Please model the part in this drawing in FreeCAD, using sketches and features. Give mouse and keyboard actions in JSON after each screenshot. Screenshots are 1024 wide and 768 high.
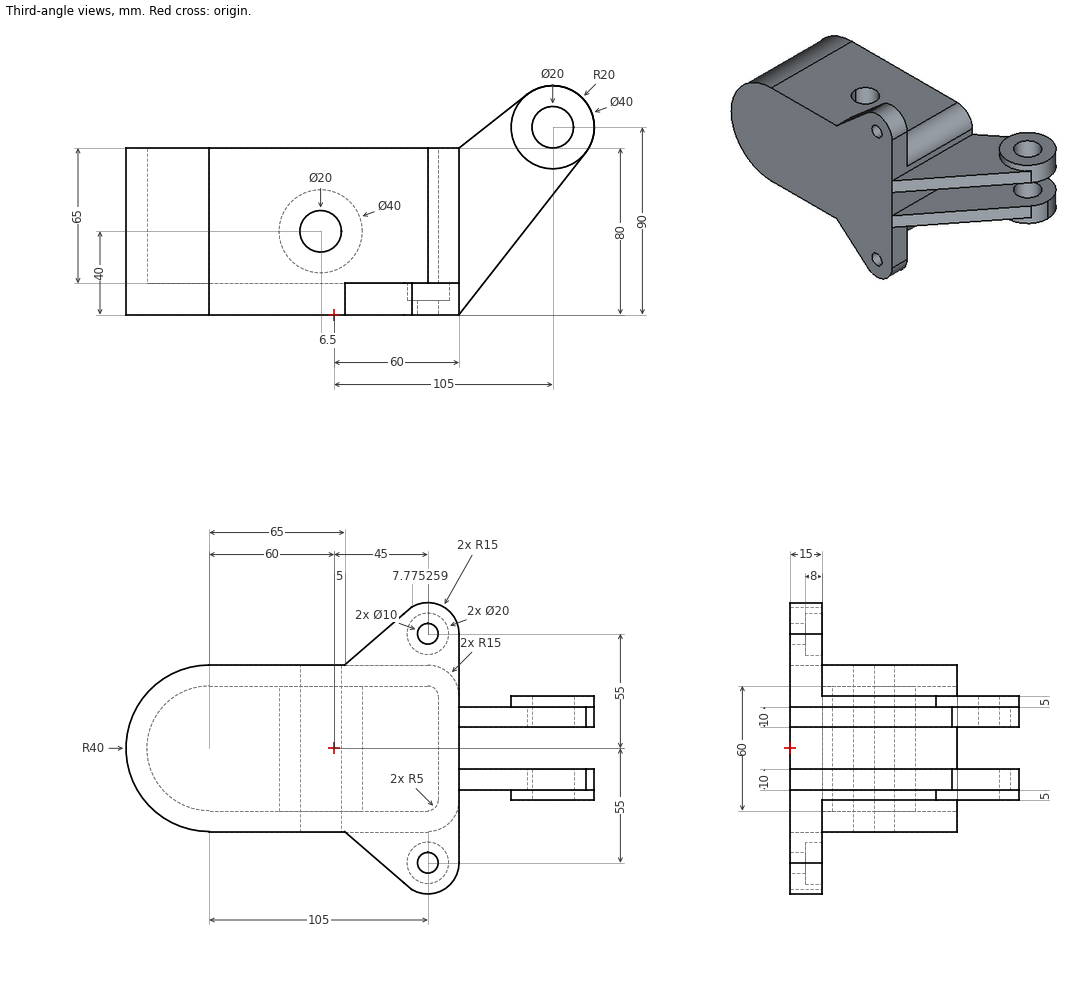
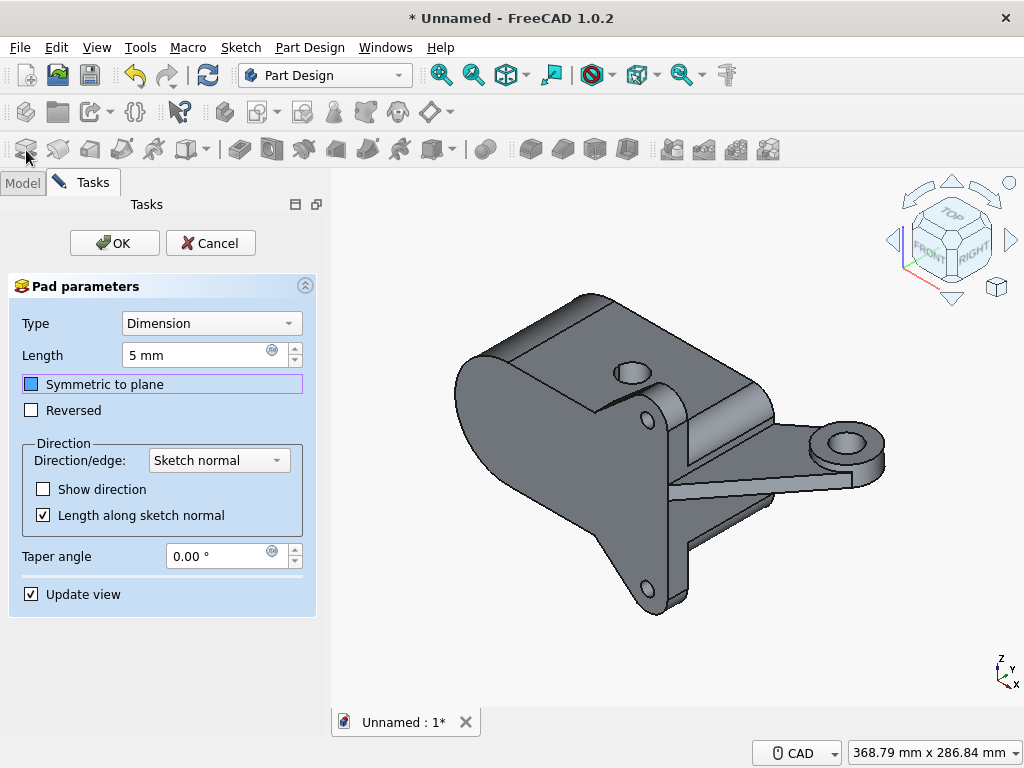
{"action": "left_click", "coordinate": [115, 243]}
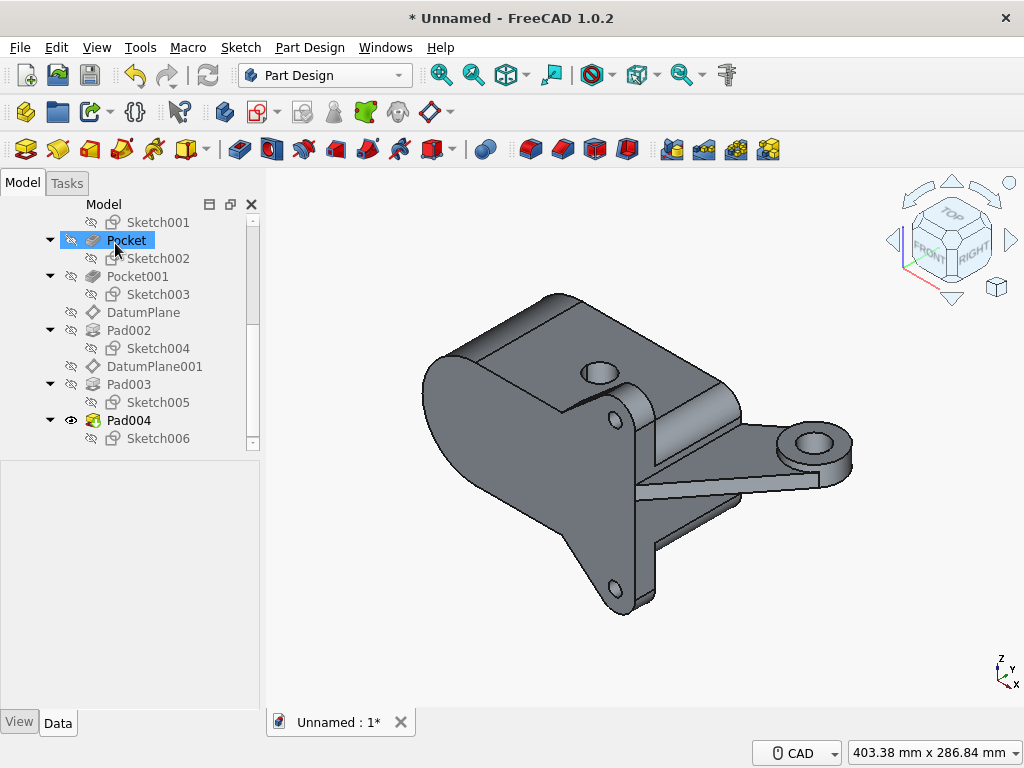
{"action": "scroll", "coordinate": [160, 326], "scroll_direction": "down", "scroll_amount": 3}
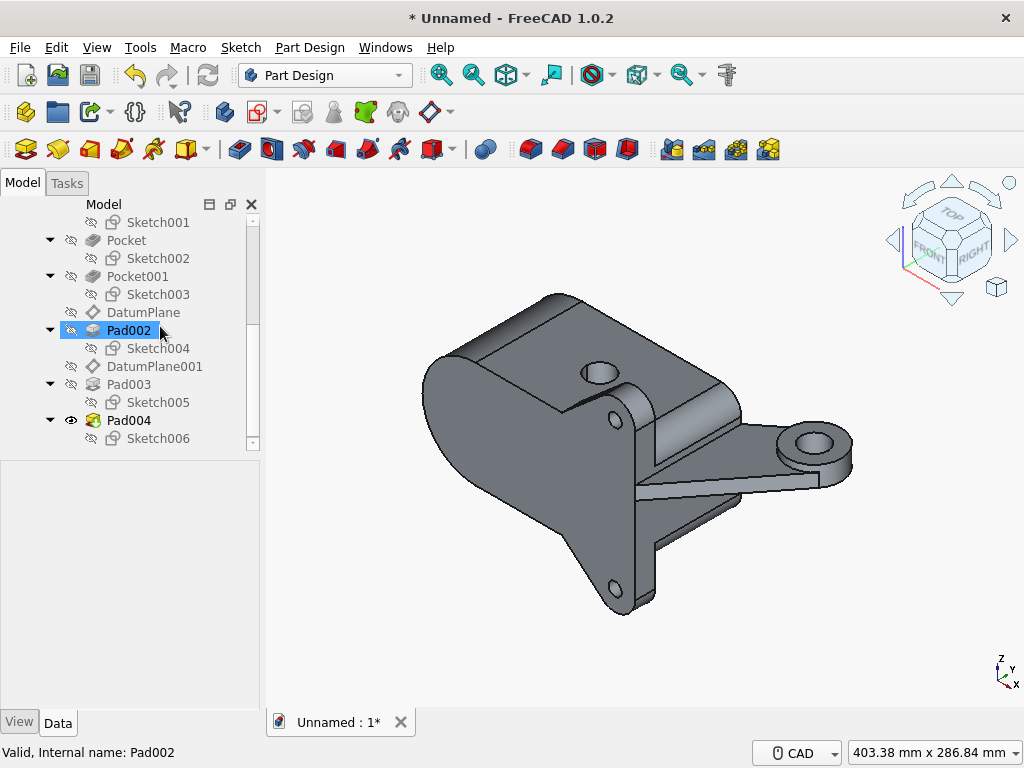
{"action": "scroll", "coordinate": [160, 326], "scroll_direction": "up", "scroll_amount": 15}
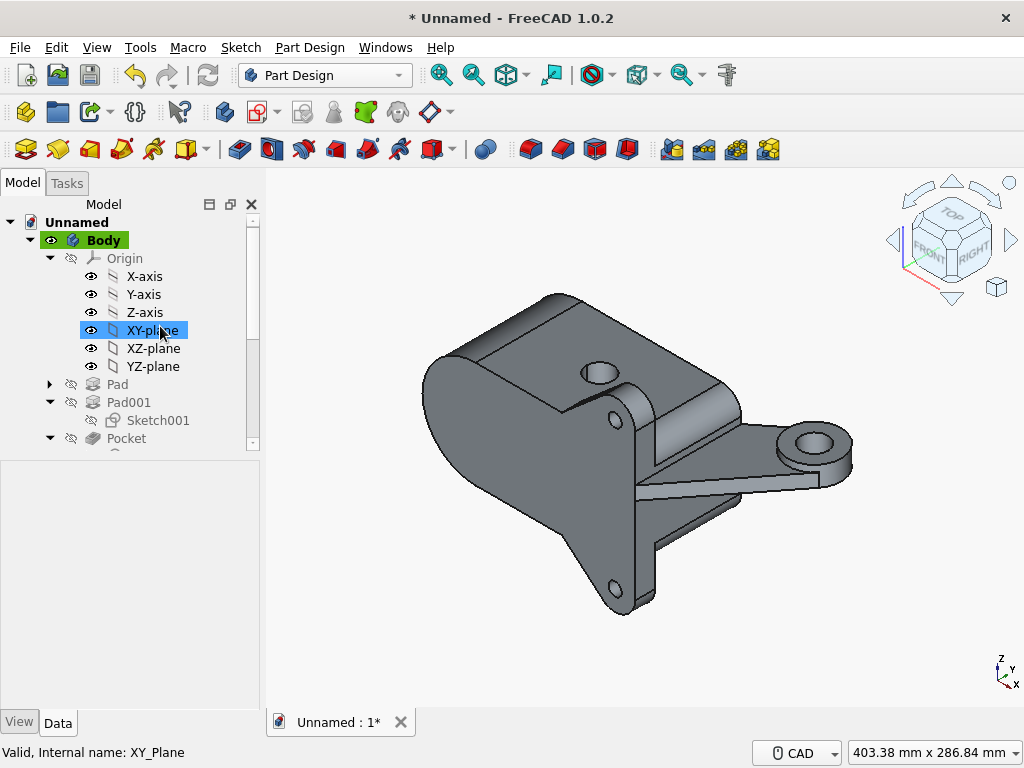
{"action": "left_click", "coordinate": [136, 330]}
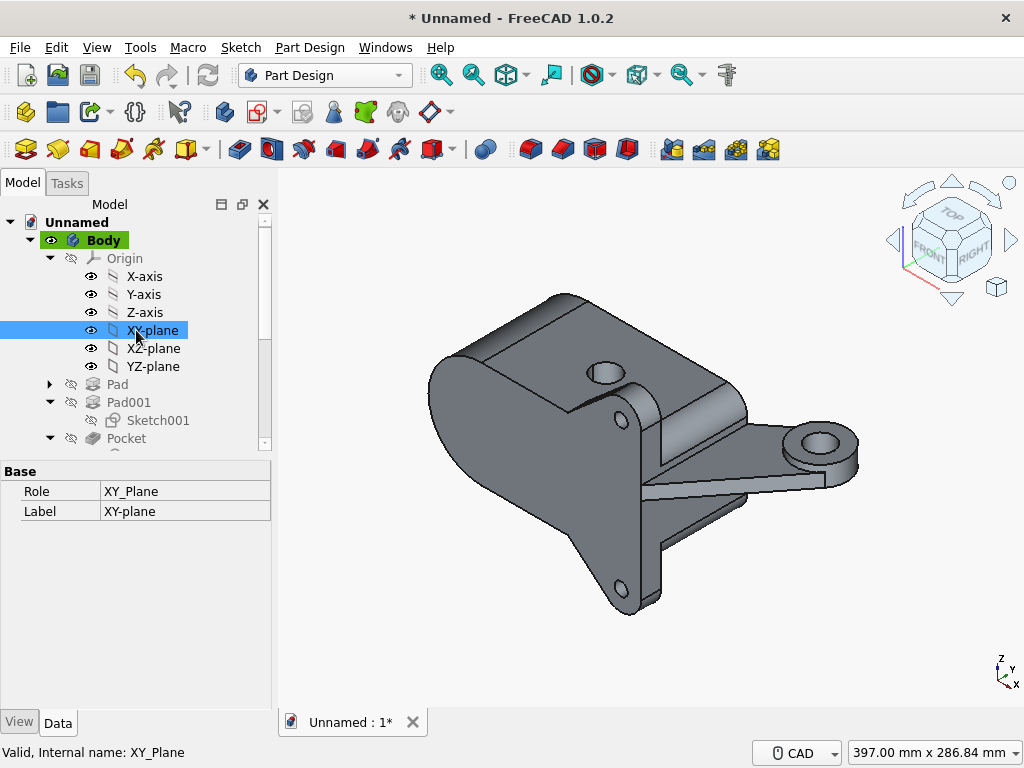
{"action": "left_click", "coordinate": [430, 112]}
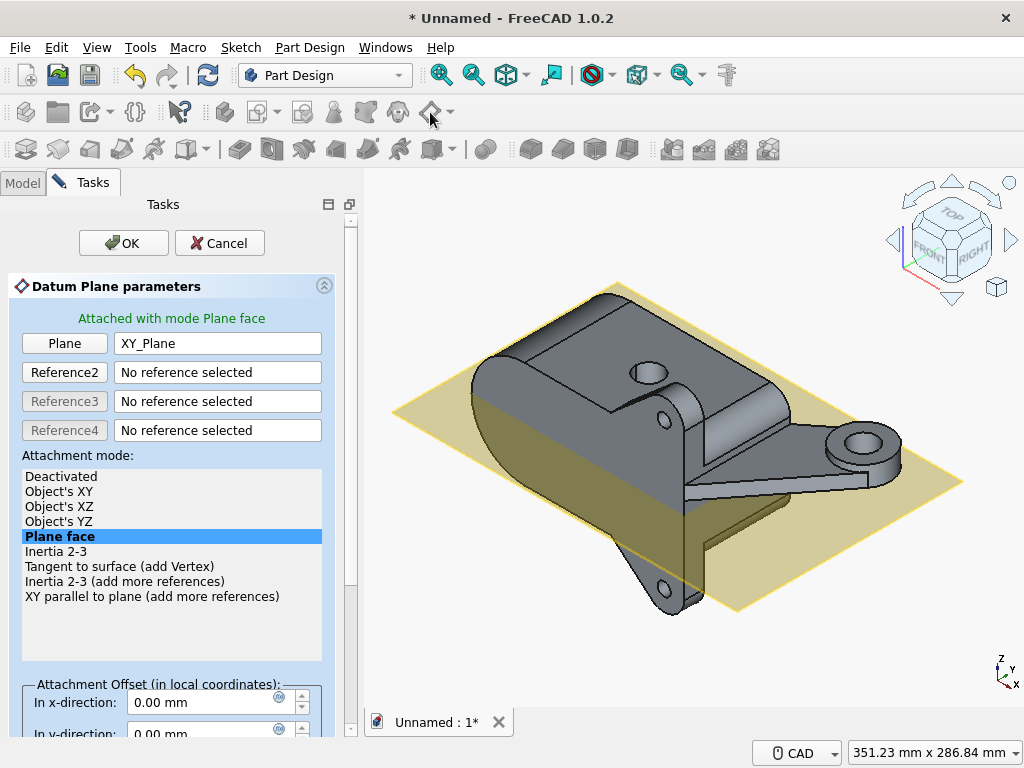
{"action": "scroll", "coordinate": [351, 475], "scroll_direction": "down", "scroll_amount": 2}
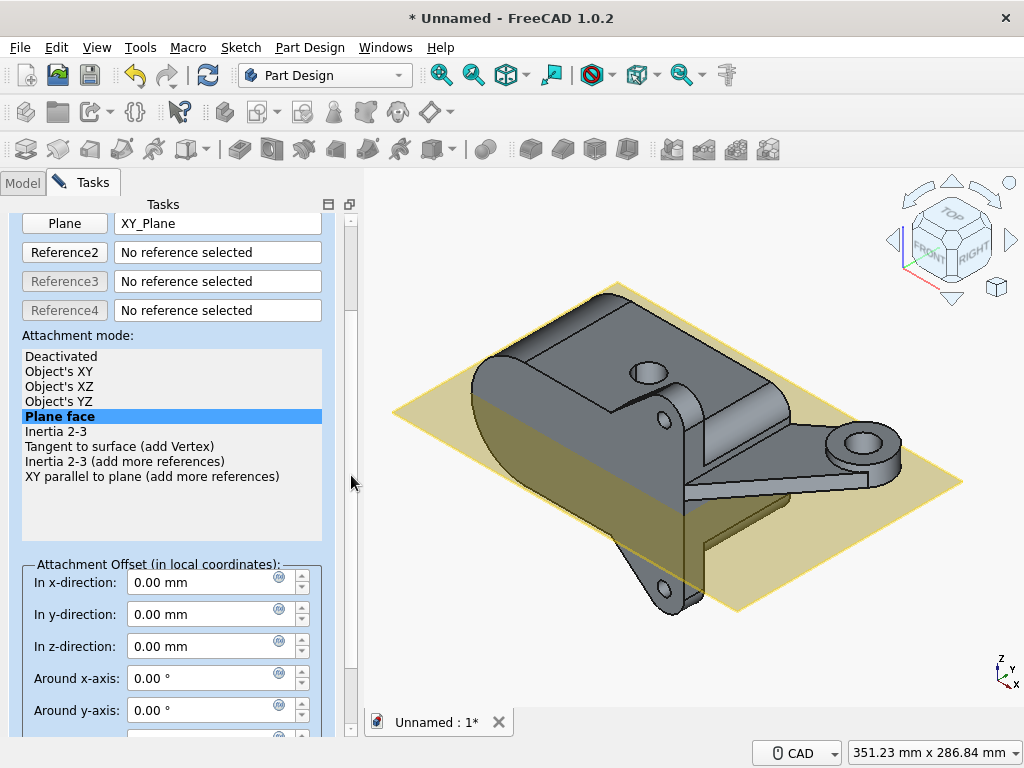
{"action": "triple_click", "coordinate": [210, 646]}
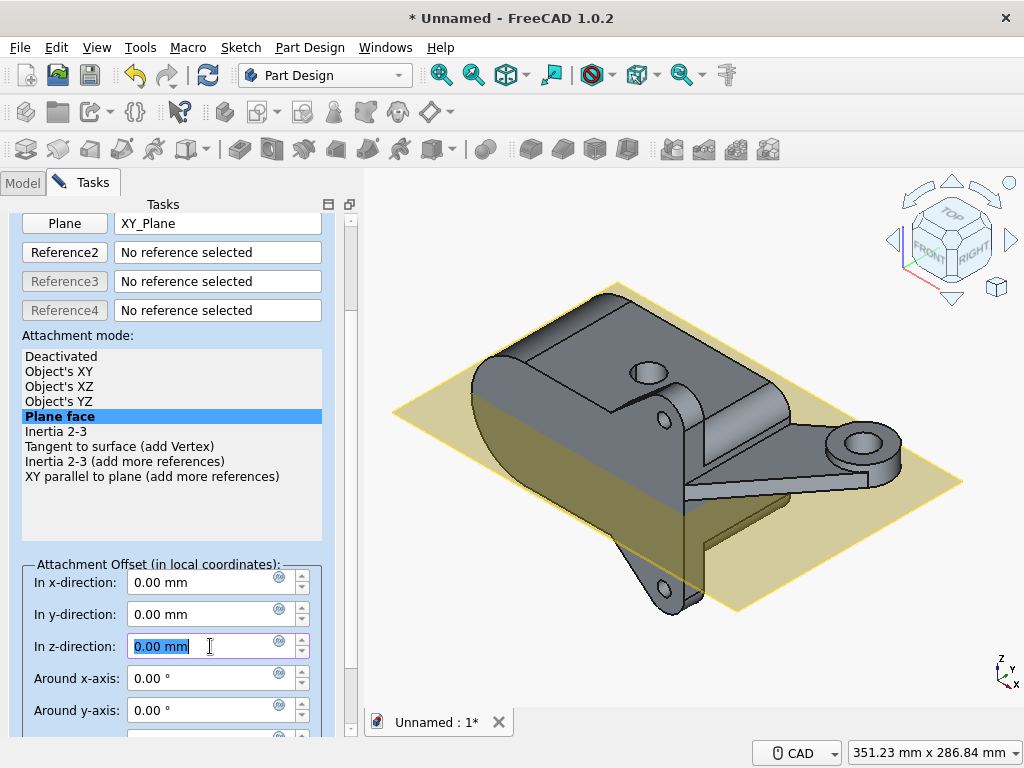
{"action": "type", "text": "-20"}
{"action": "key", "text": "Tab"}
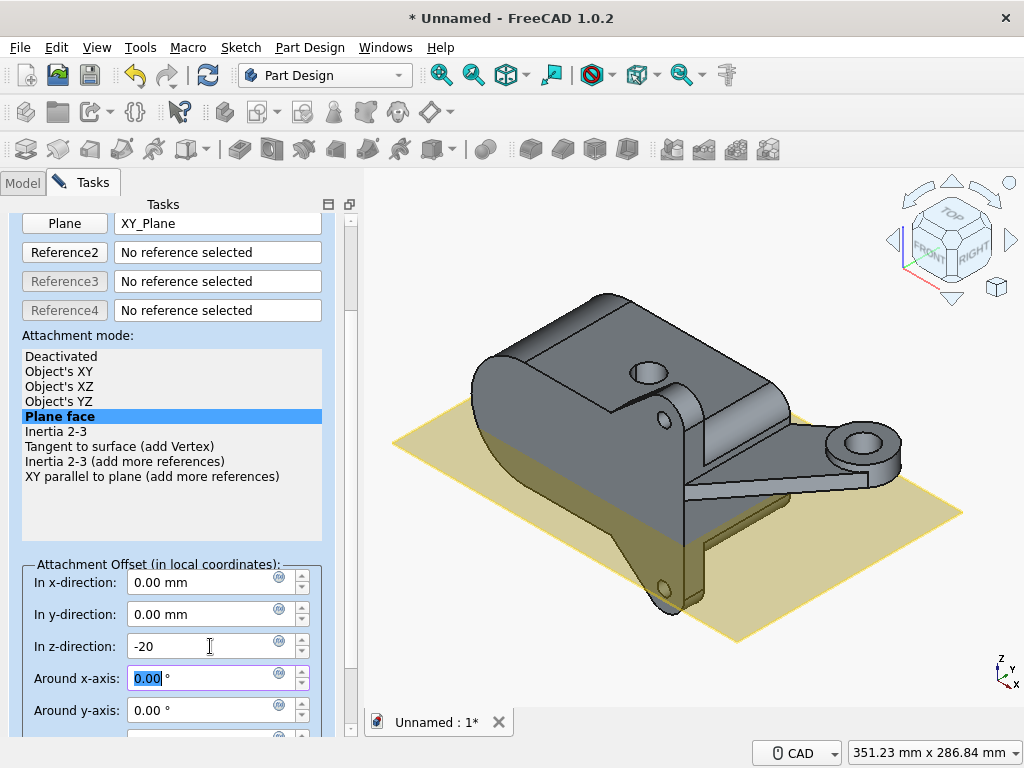
{"action": "scroll", "coordinate": [351, 475], "scroll_direction": "up", "scroll_amount": 3}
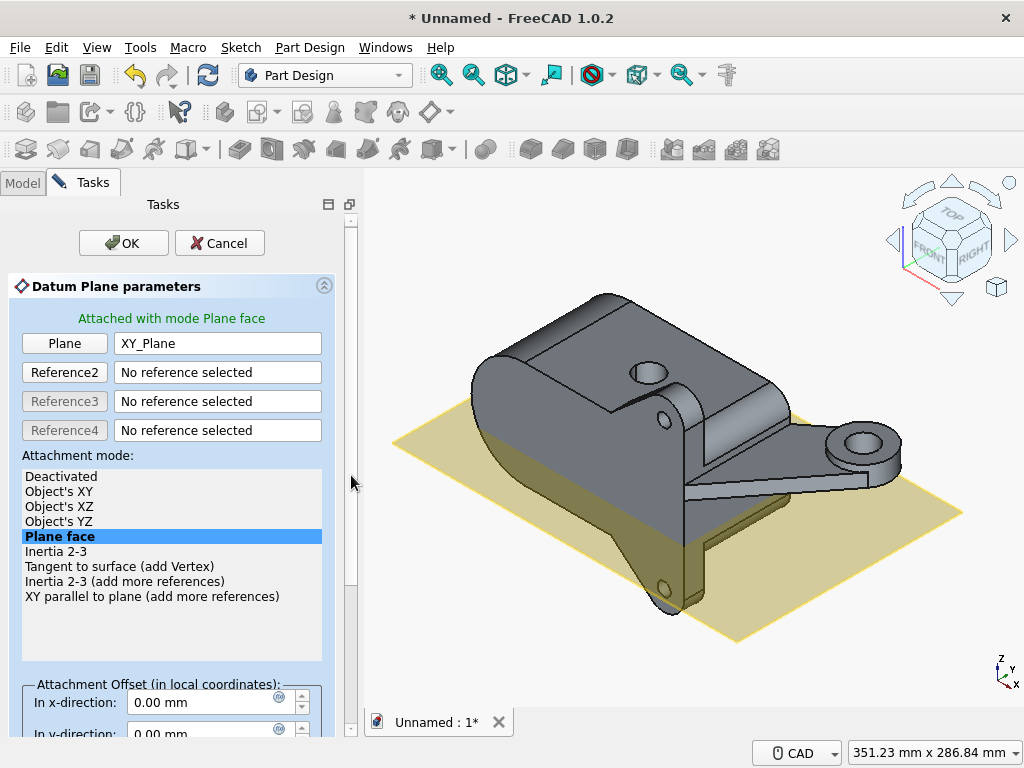
{"action": "left_click", "coordinate": [124, 243]}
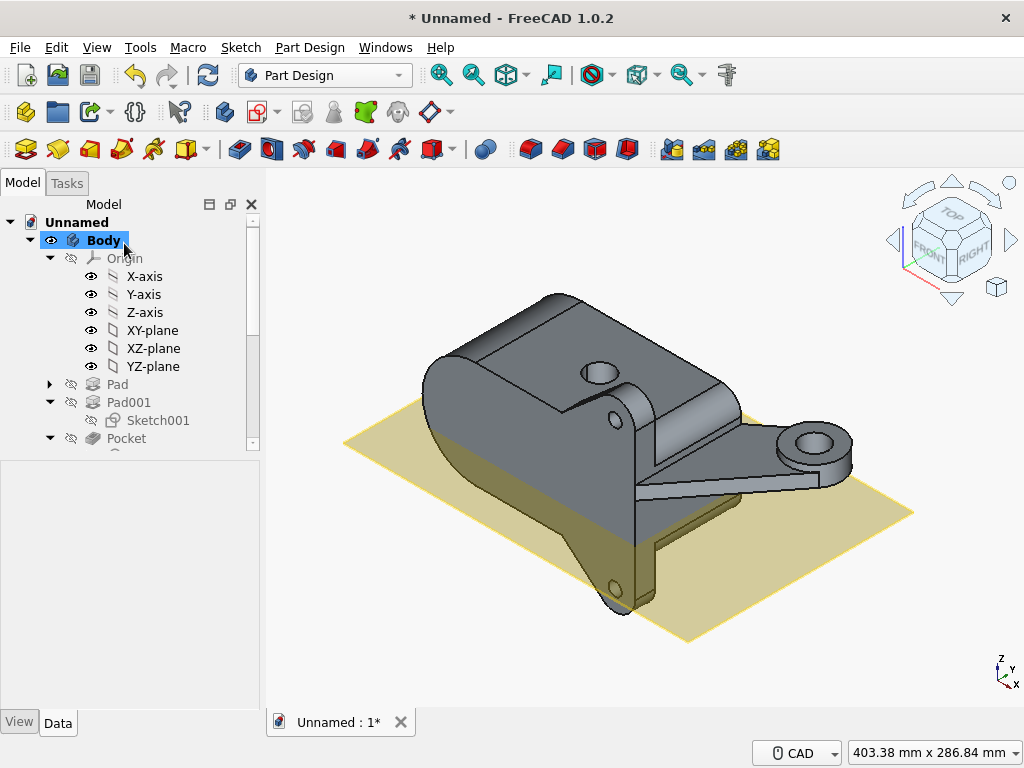
{"action": "scroll", "coordinate": [100, 326], "scroll_direction": "down", "scroll_amount": 3}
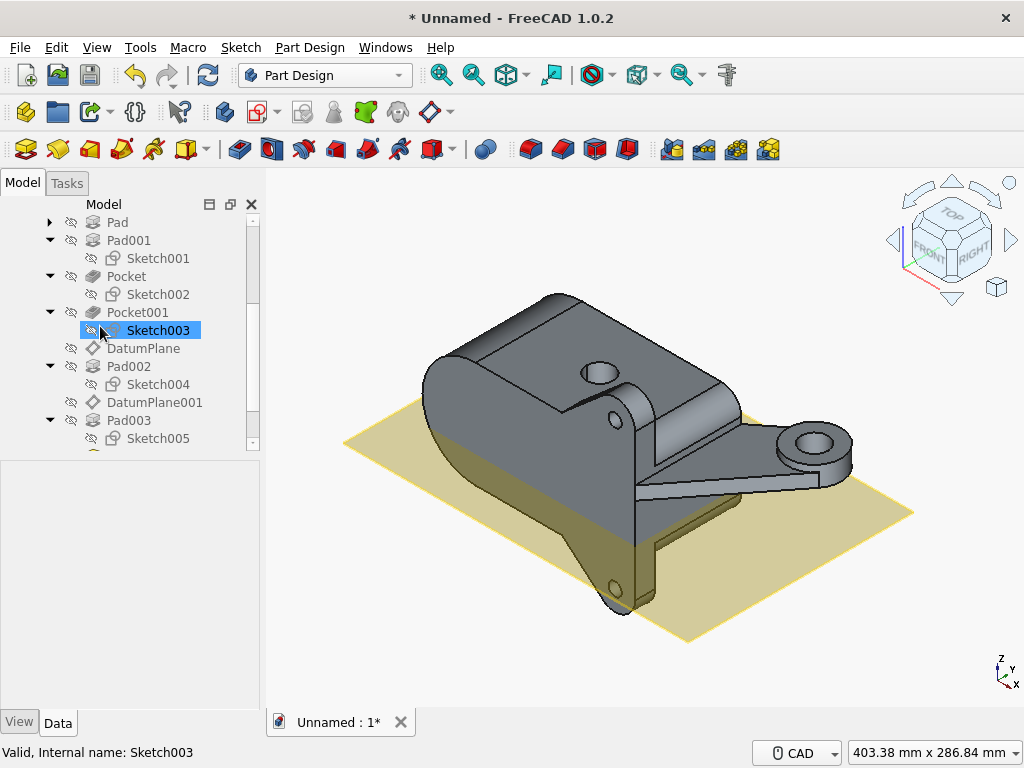
{"action": "scroll", "coordinate": [140, 326], "scroll_direction": "up", "scroll_amount": 15}